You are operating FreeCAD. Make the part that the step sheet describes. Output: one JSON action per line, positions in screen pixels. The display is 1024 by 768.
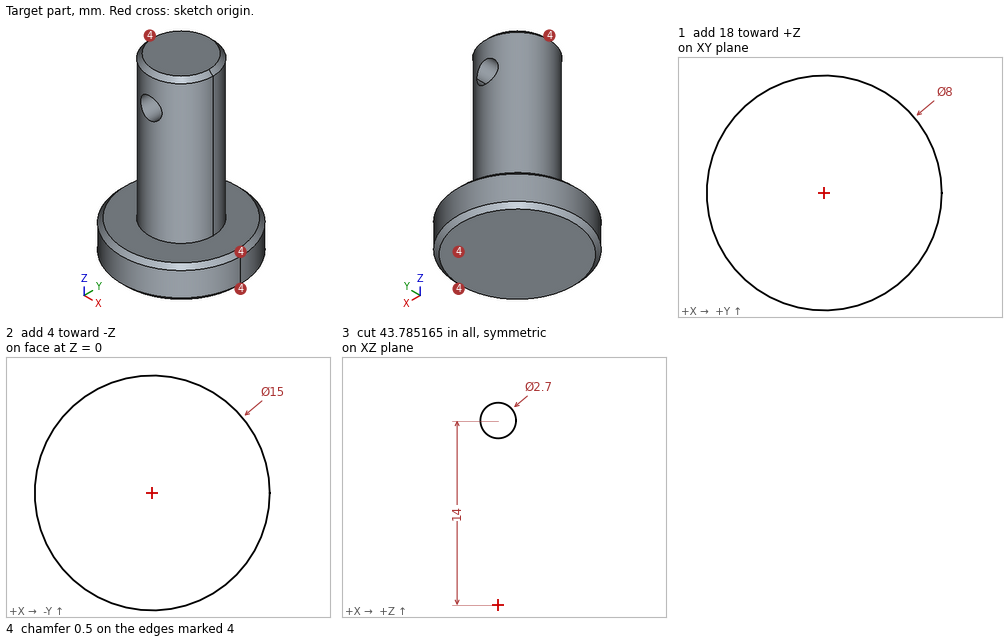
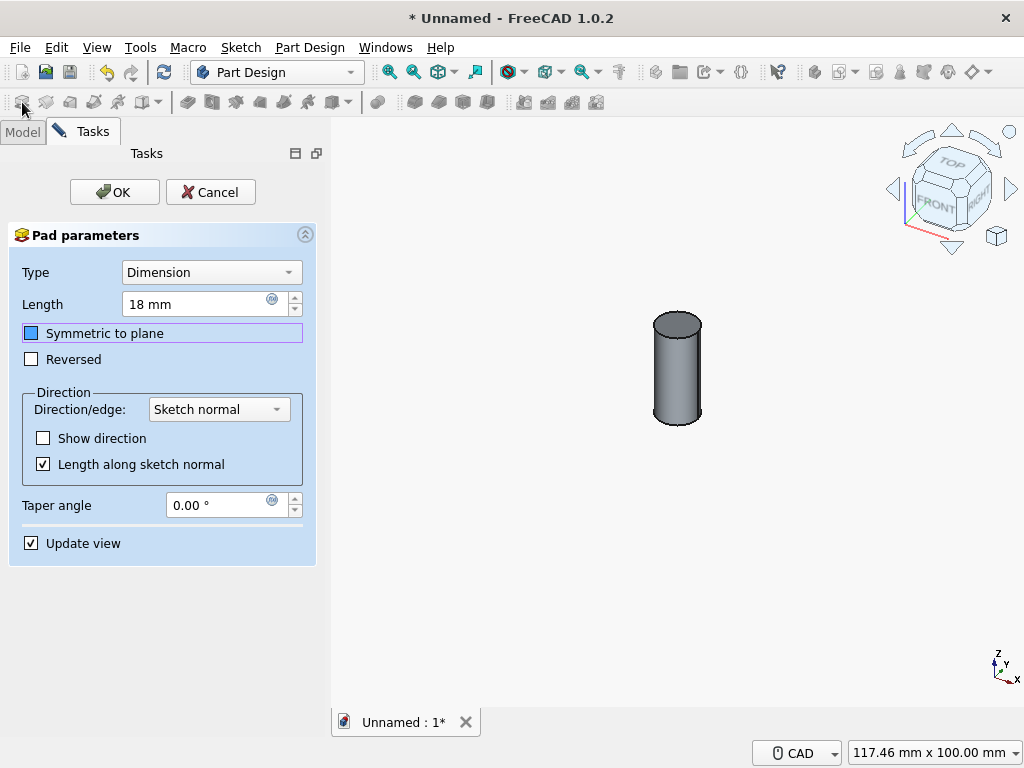
{"action": "left_click", "coordinate": [115, 192]}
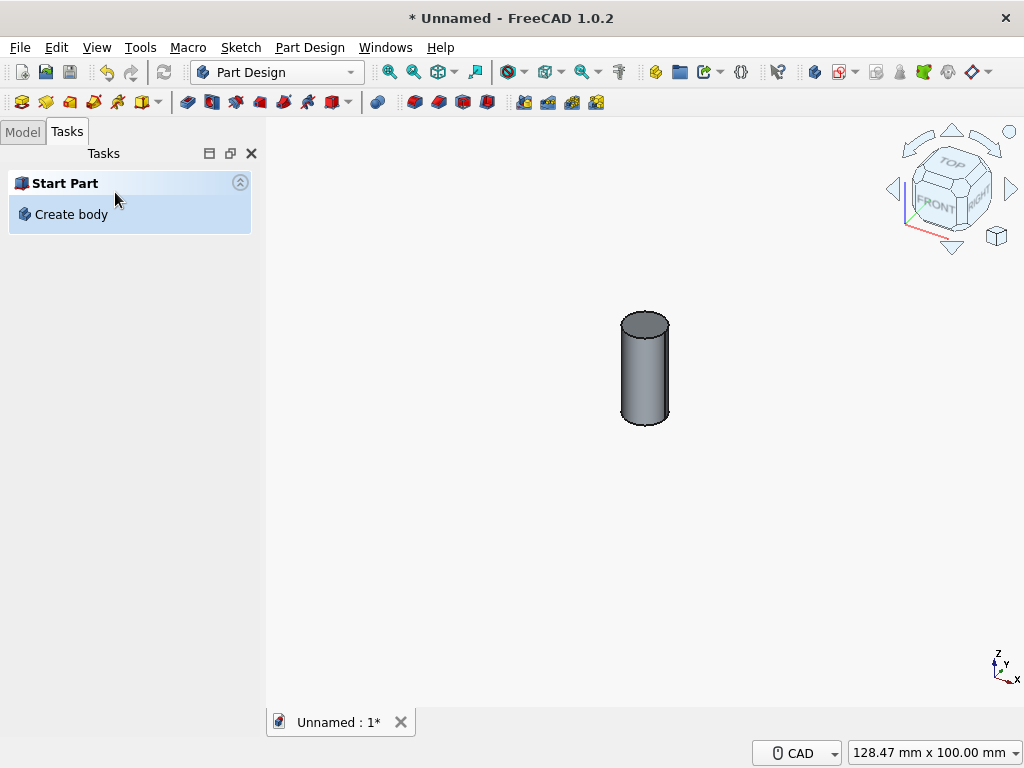
{"action": "left_click", "coordinate": [390, 72]}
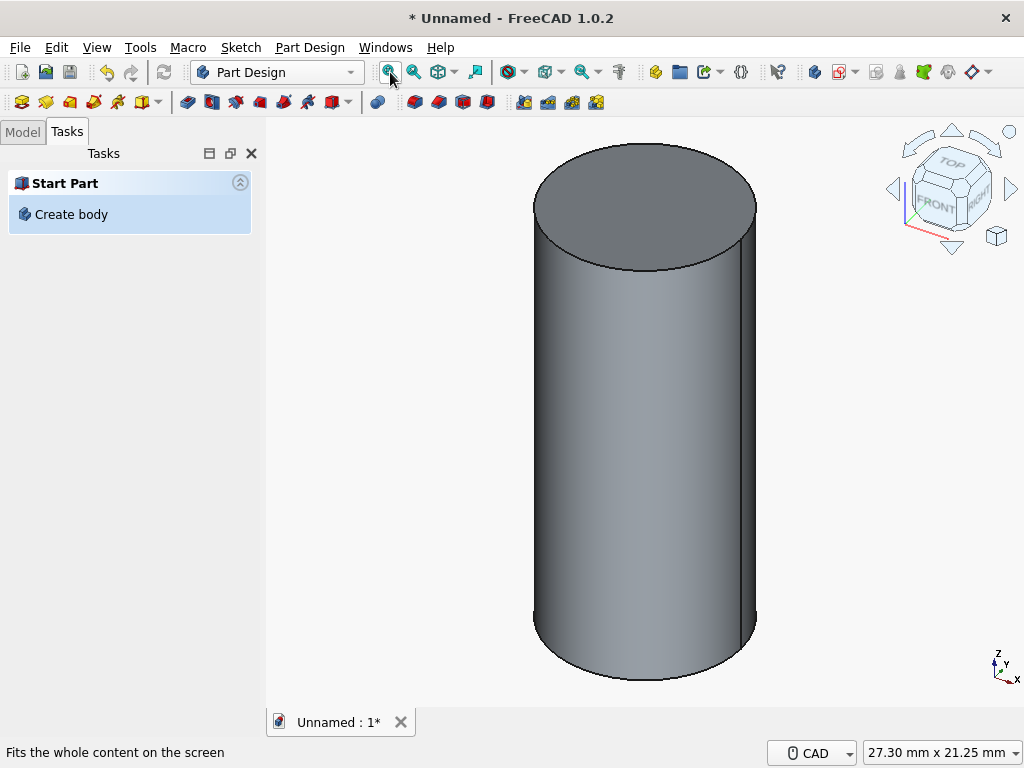
{"action": "key", "text": "5"}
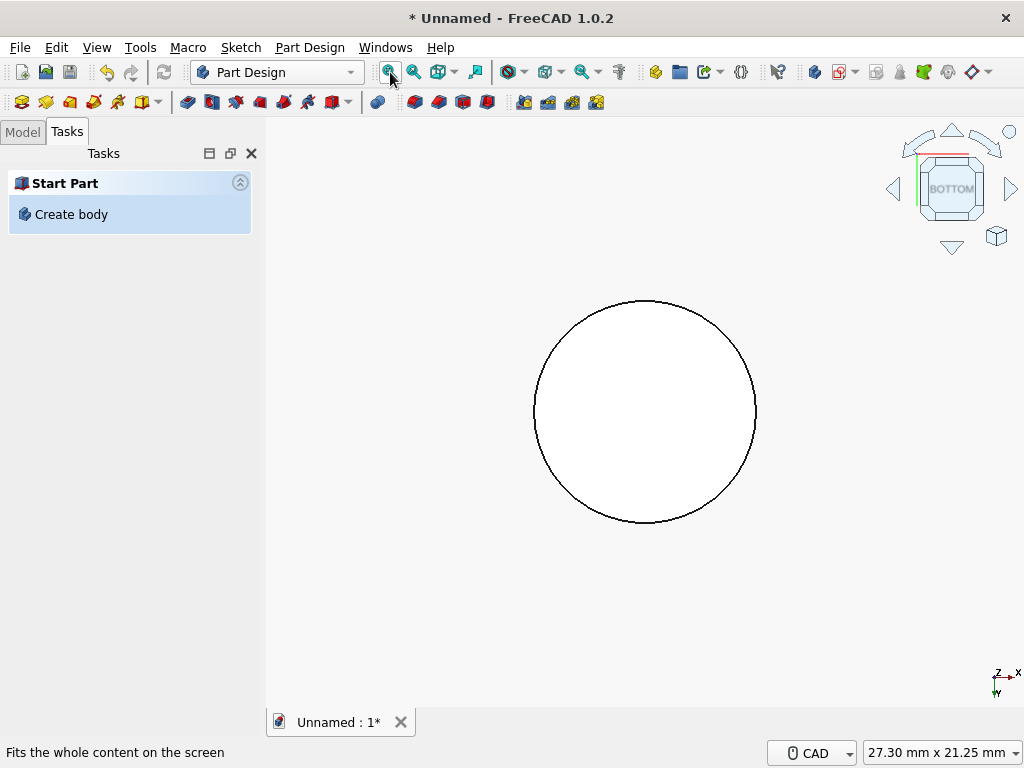
{"action": "left_click", "coordinate": [390, 72]}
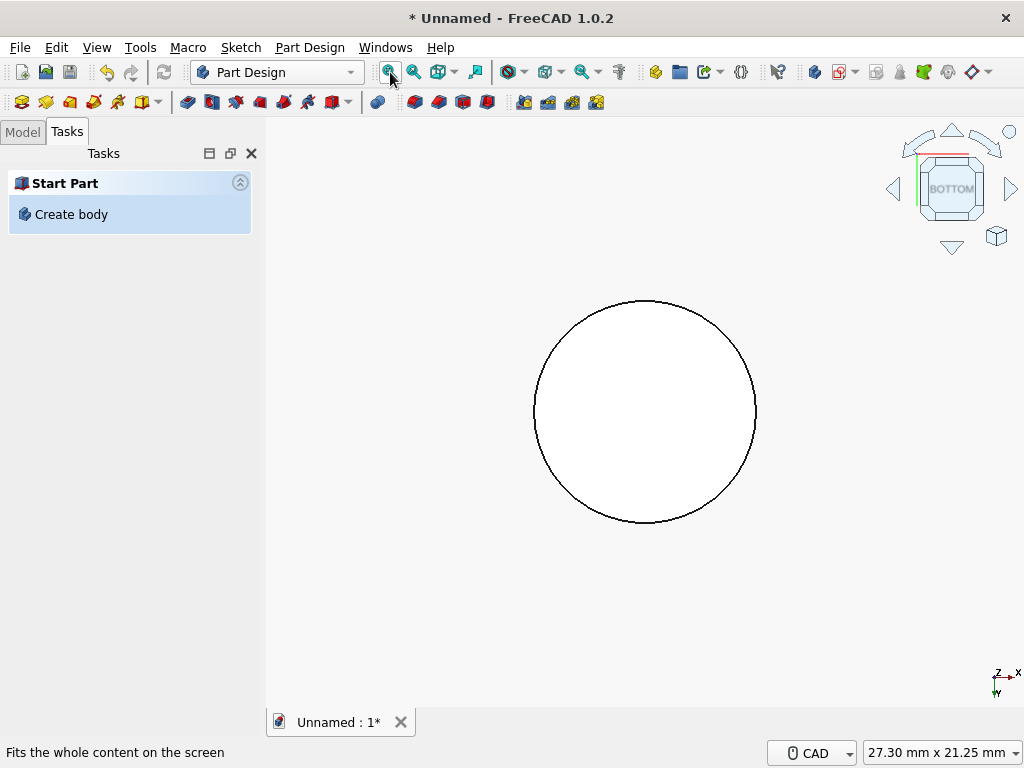
{"action": "left_click", "coordinate": [645, 411]}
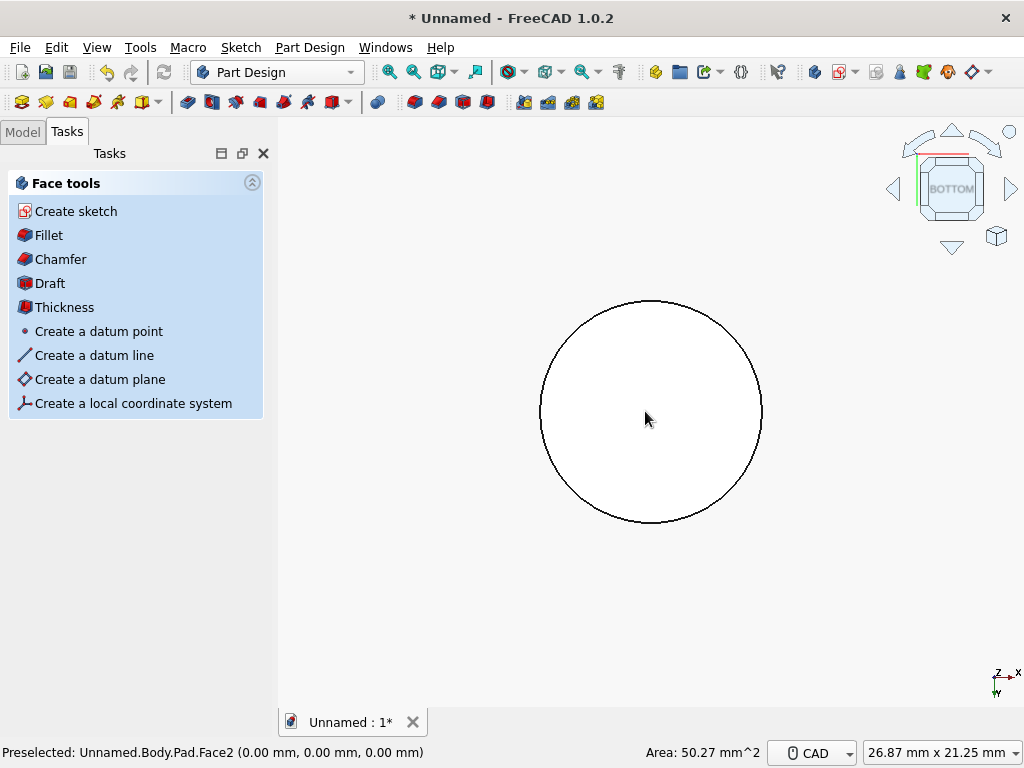
{"action": "left_click", "coordinate": [840, 72]}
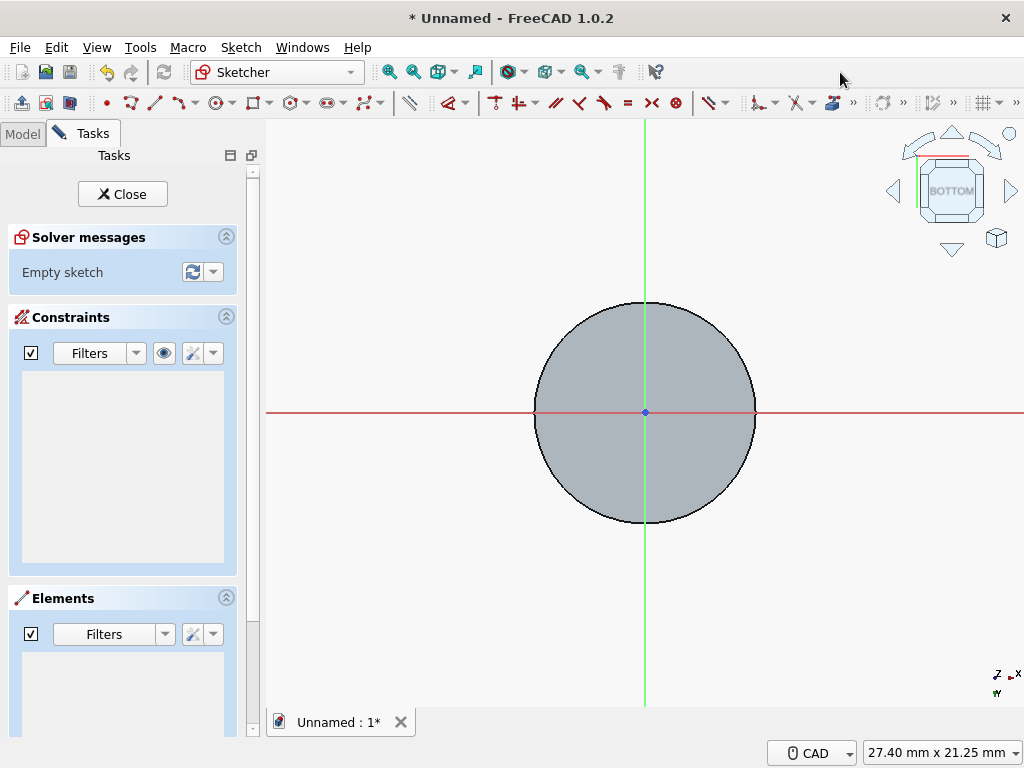
{"action": "scroll", "coordinate": [294, 413], "scroll_direction": "down", "scroll_amount": 1}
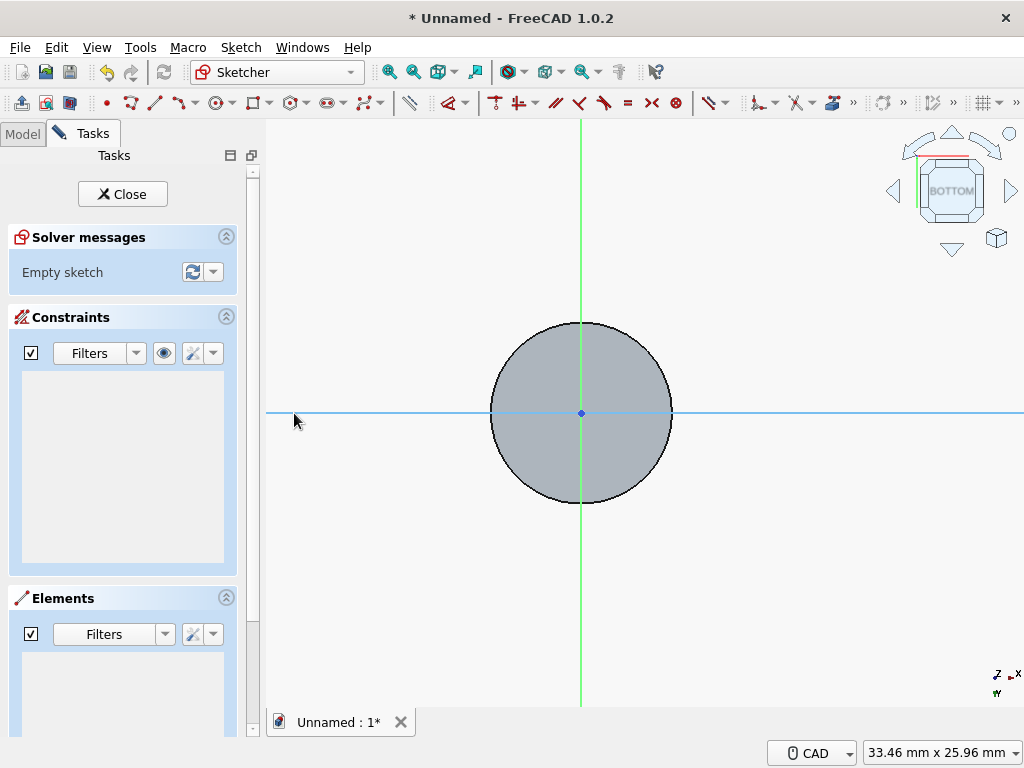
{"action": "left_click", "coordinate": [216, 104]}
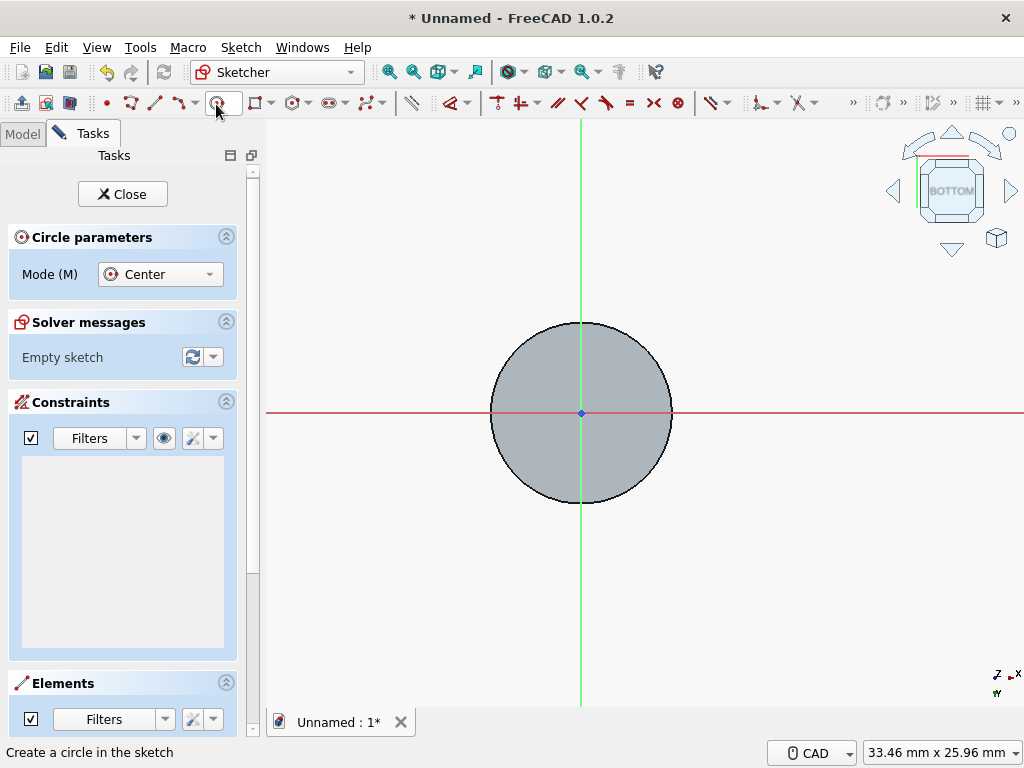
{"action": "left_click", "coordinate": [581, 413]}
{"action": "left_click", "coordinate": [702, 293]}
{"action": "key", "text": "Escape"}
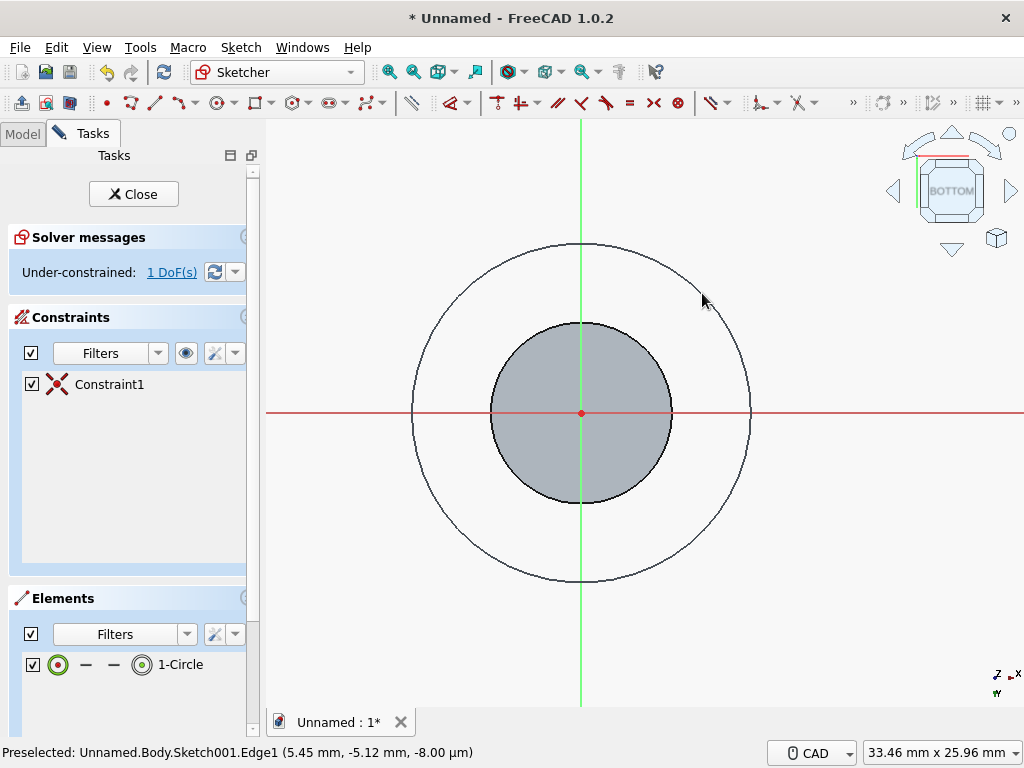
{"action": "left_click", "coordinate": [450, 104]}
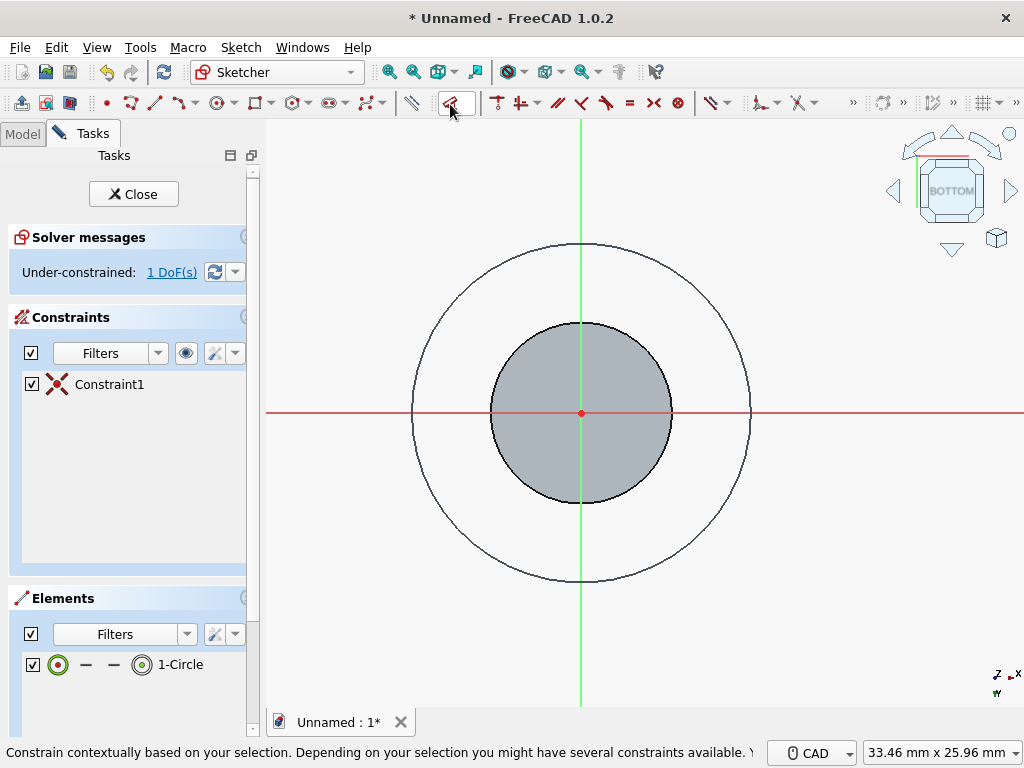
{"action": "left_click", "coordinate": [701, 293]}
{"action": "left_click", "coordinate": [724, 270]}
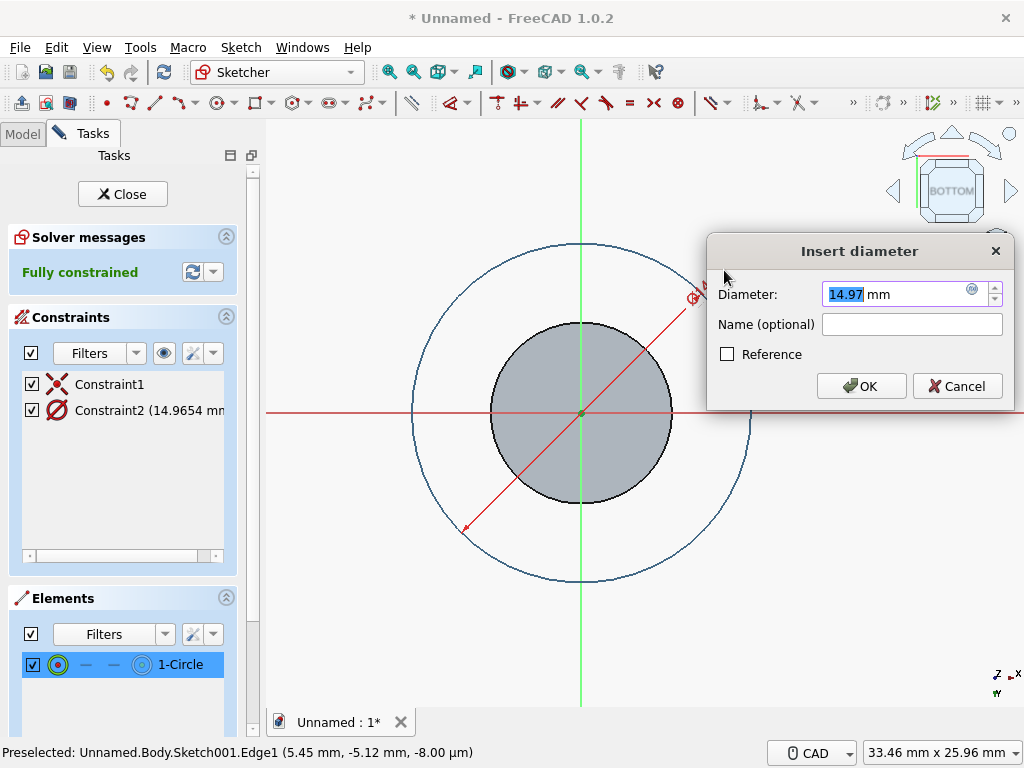
{"action": "type", "text": "15"}
{"action": "key", "text": "Return"}
{"action": "key", "text": "Escape"}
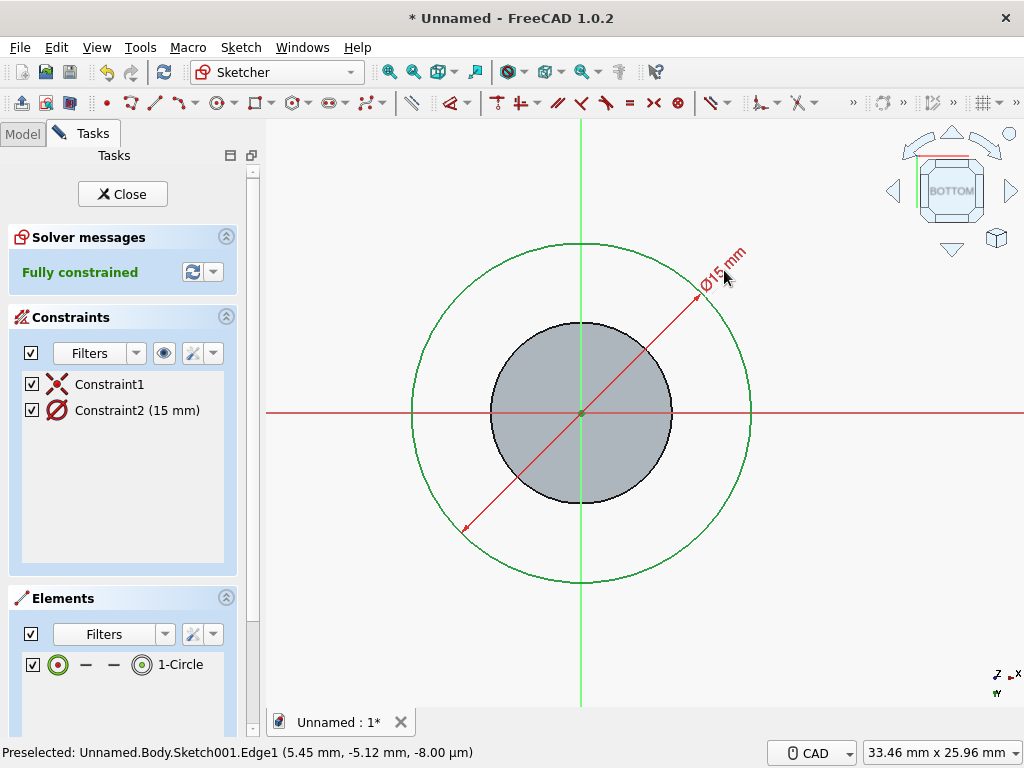
{"action": "left_click", "coordinate": [123, 194]}